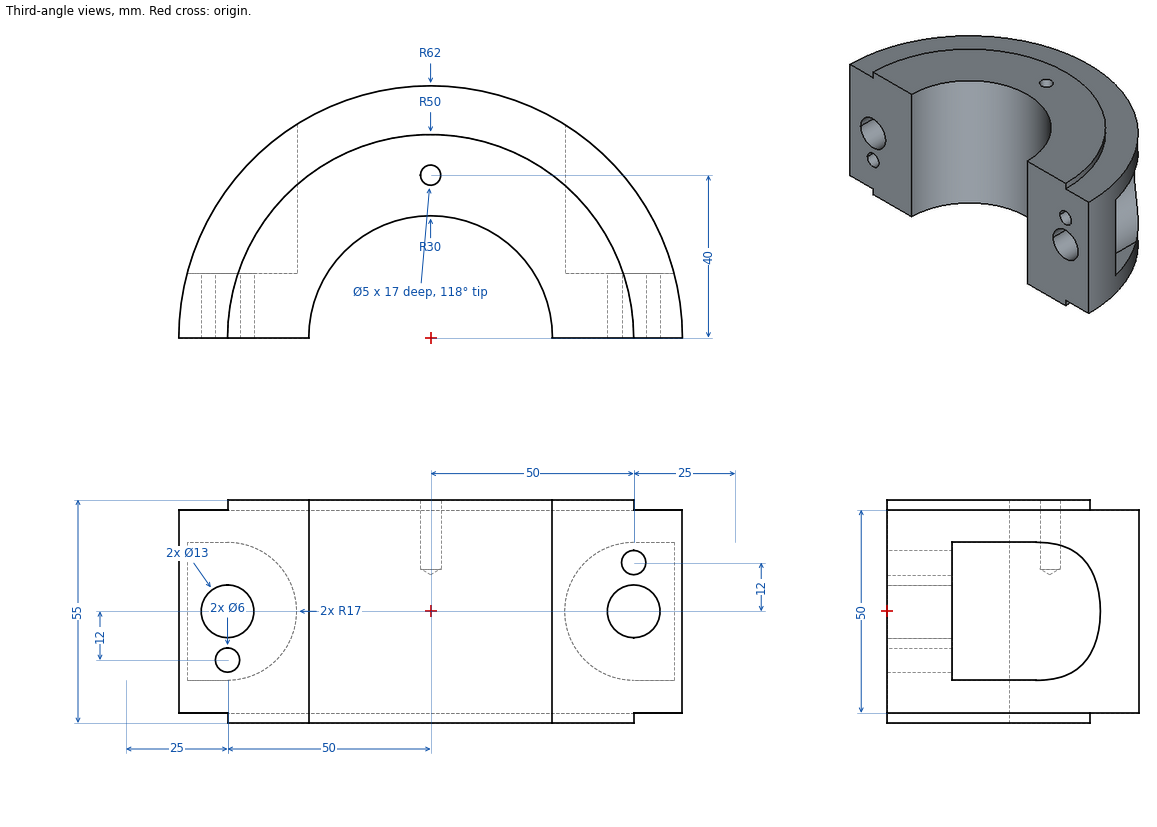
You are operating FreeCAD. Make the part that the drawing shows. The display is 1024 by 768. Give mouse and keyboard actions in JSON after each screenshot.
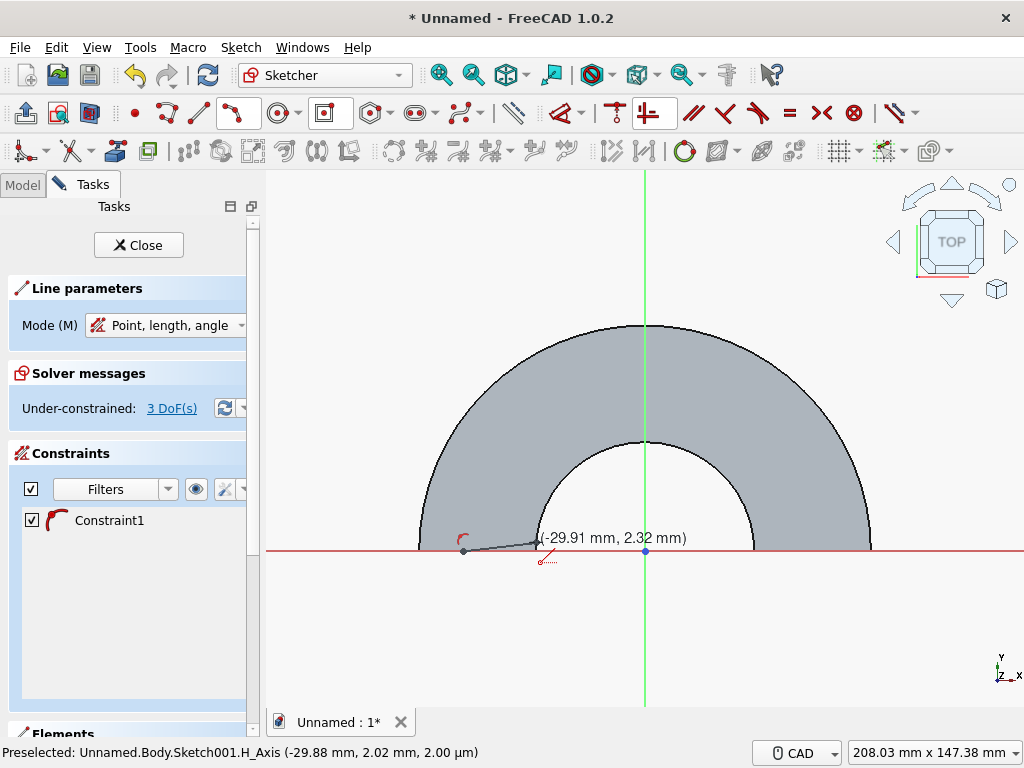
{"action": "left_click", "coordinate": [754, 551]}
{"action": "left_click", "coordinate": [827, 542]}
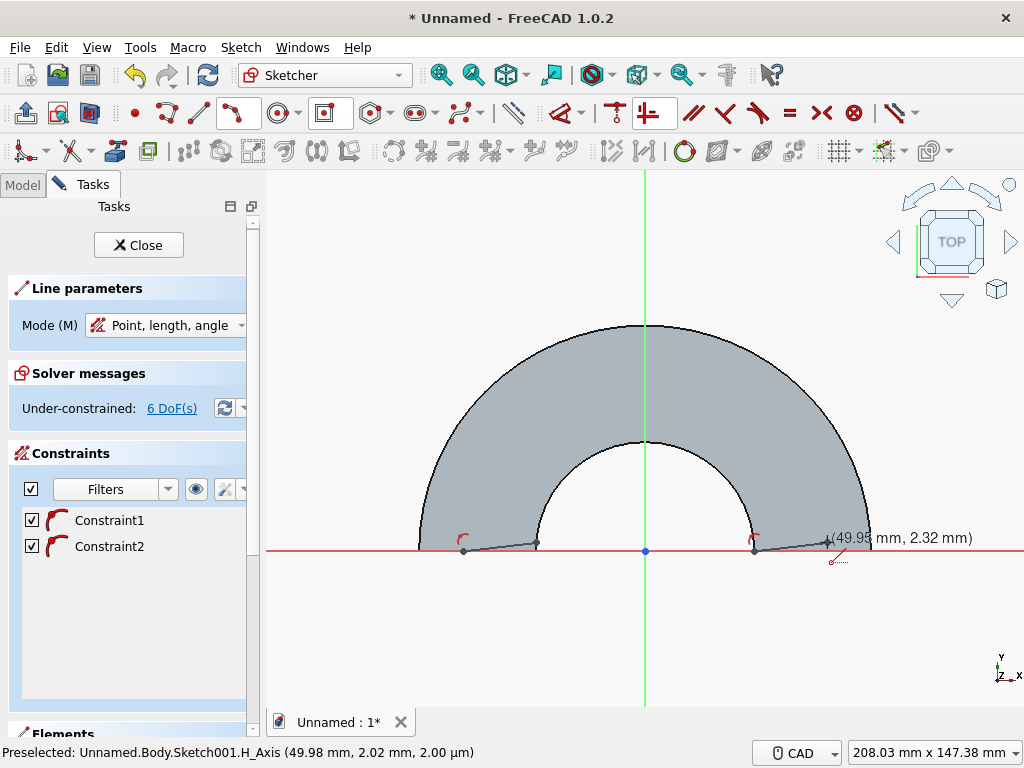
{"action": "left_click", "coordinate": [232, 114]}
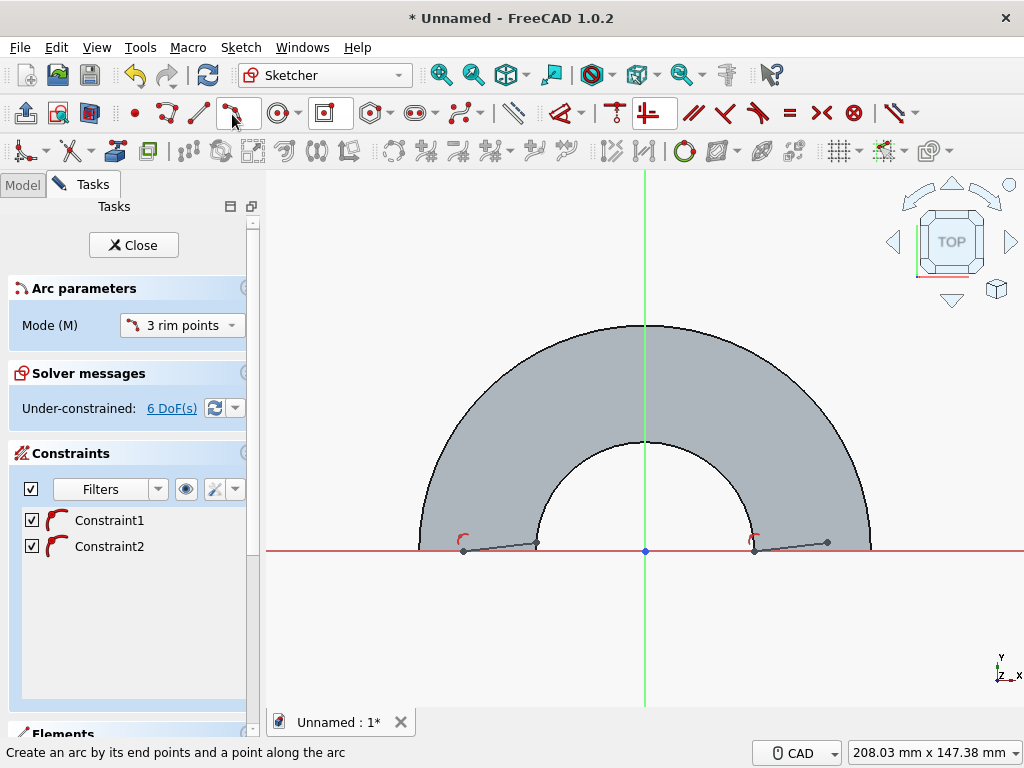
{"action": "left_click", "coordinate": [536, 543]}
{"action": "left_click", "coordinate": [754, 551]}
{"action": "left_click", "coordinate": [679, 447]}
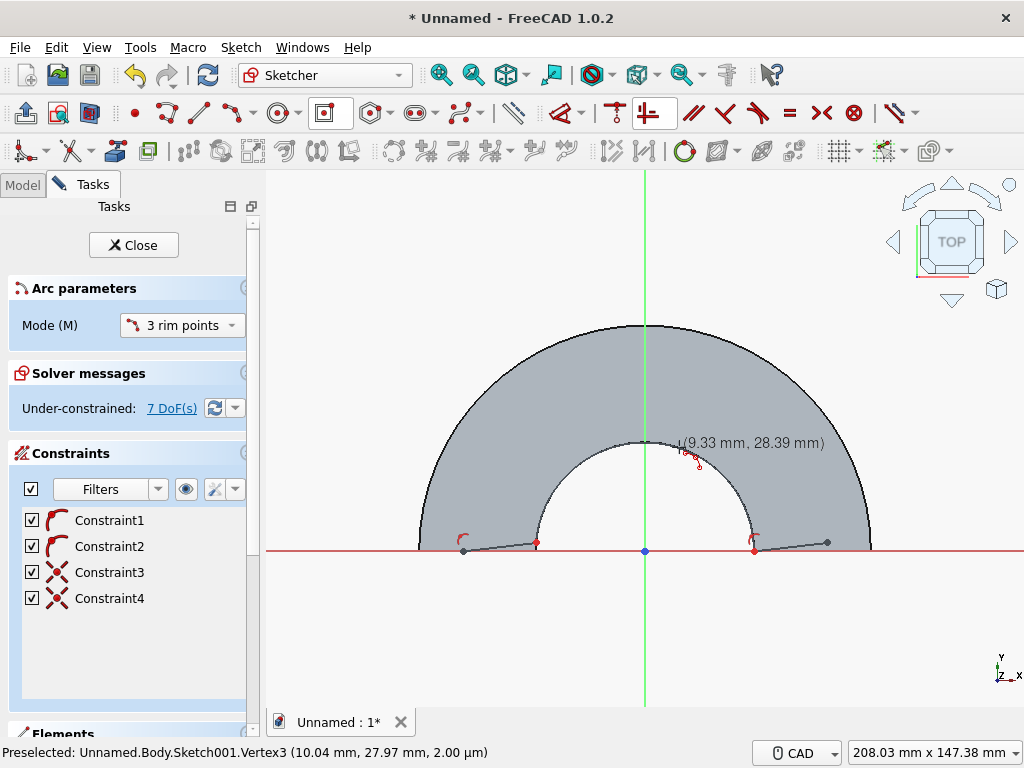
{"action": "left_click", "coordinate": [827, 543]}
{"action": "left_click", "coordinate": [463, 551]}
{"action": "left_click", "coordinate": [701, 378]}
{"action": "key", "text": "Escape"}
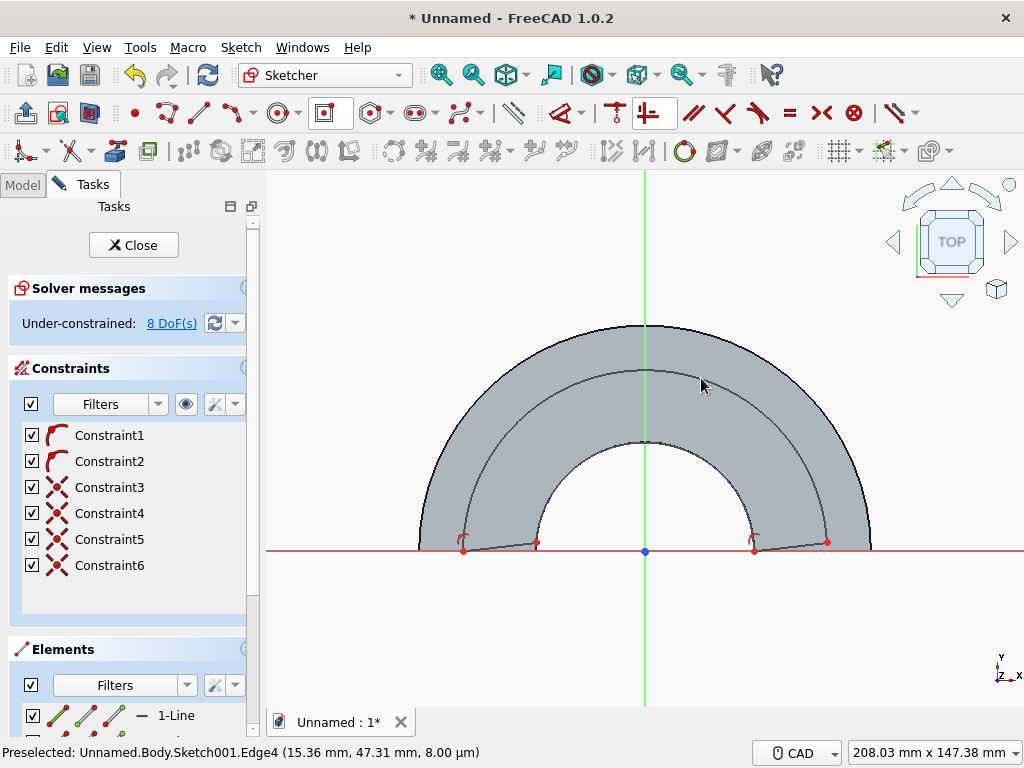
{"action": "left_click", "coordinate": [485, 549]}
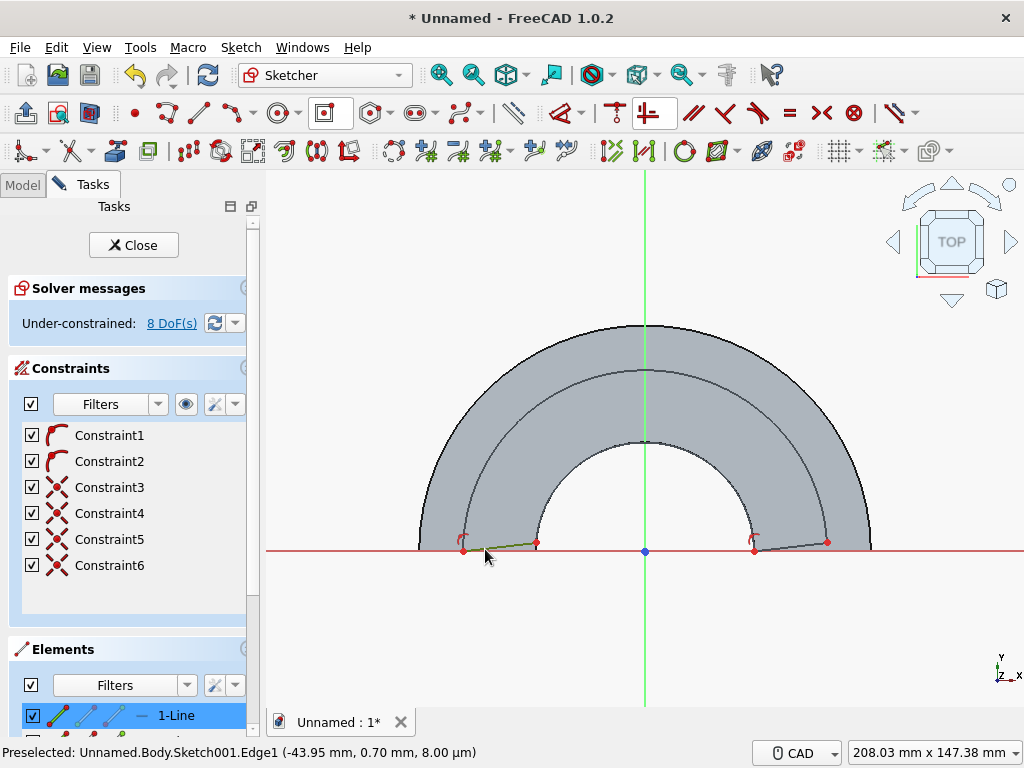
{"action": "key", "text": "h"}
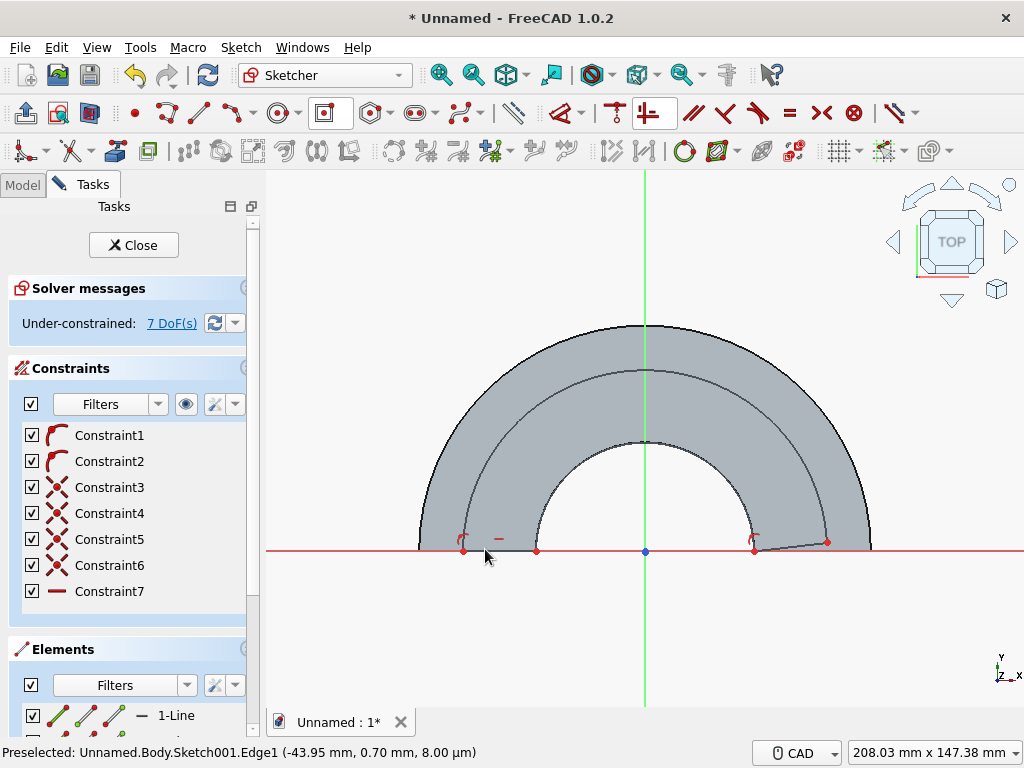
{"action": "left_click", "coordinate": [776, 549]}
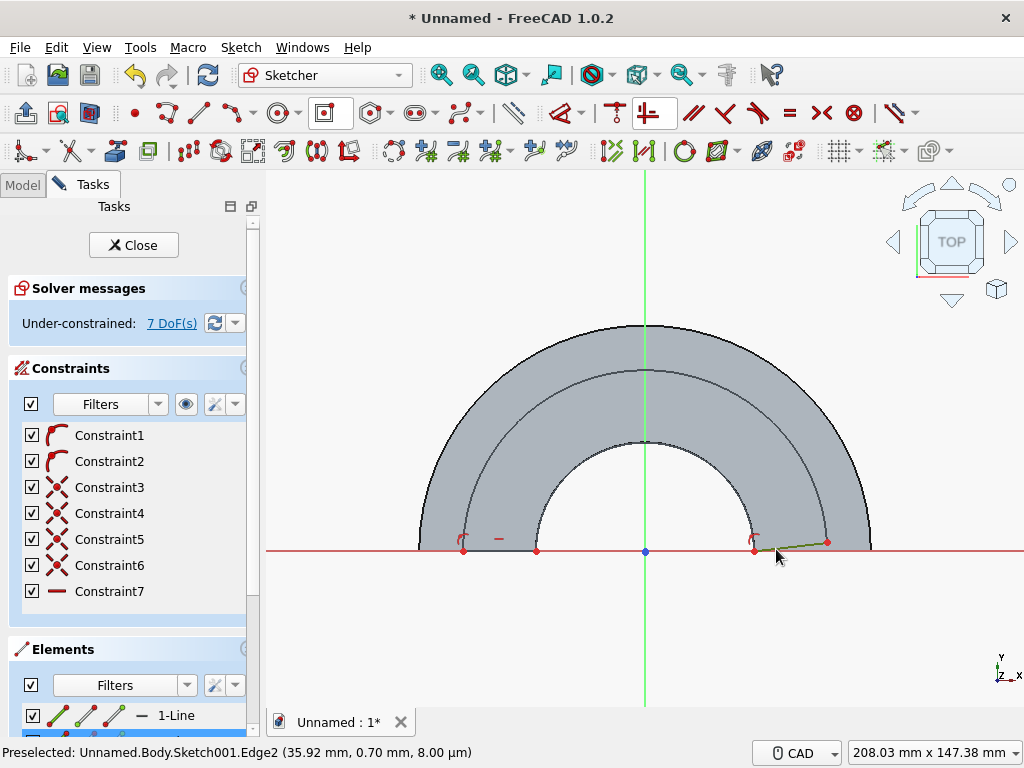
{"action": "key", "text": "h"}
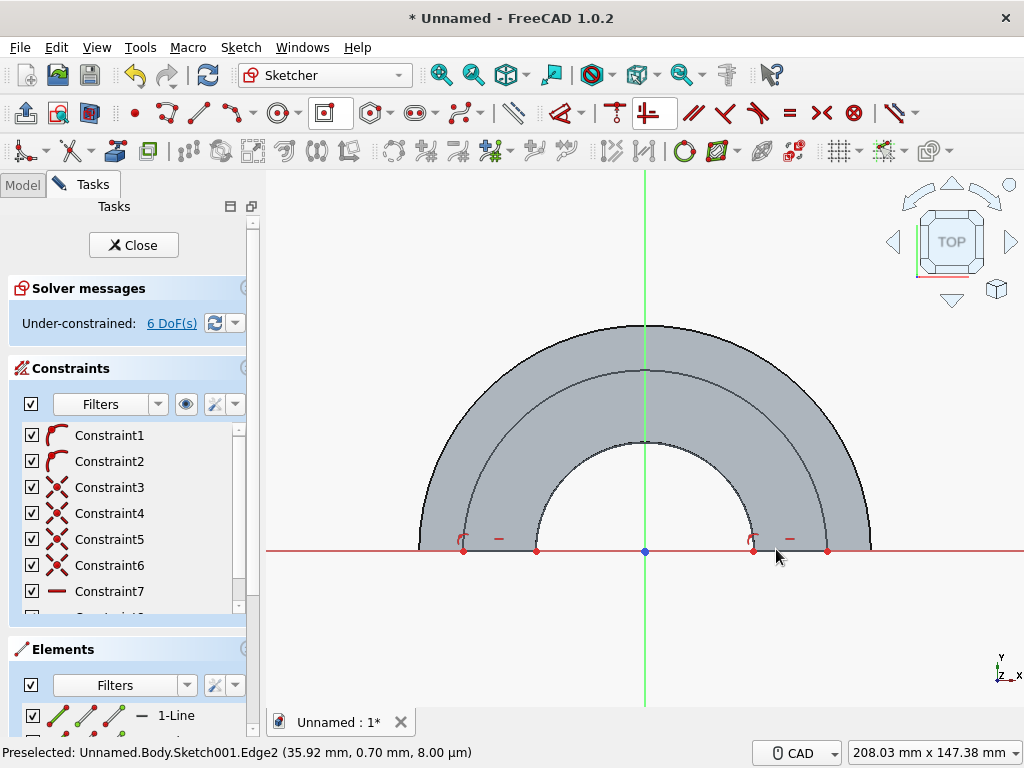
{"action": "left_click", "coordinate": [709, 463]}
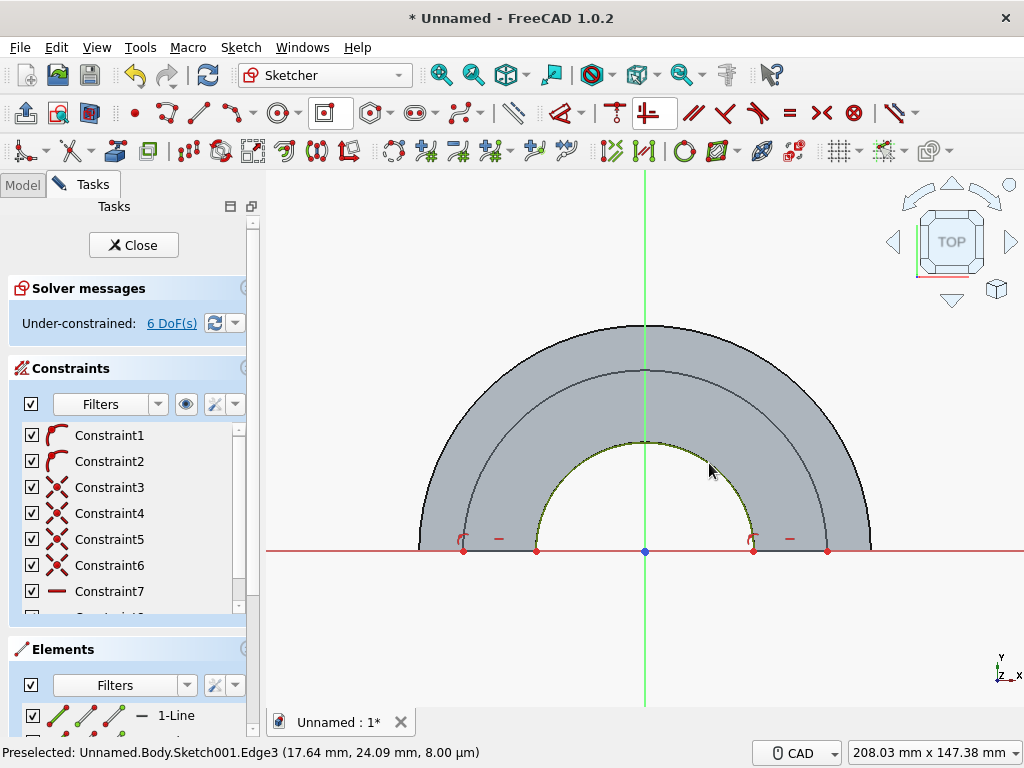
{"action": "left_click", "coordinate": [752, 405]}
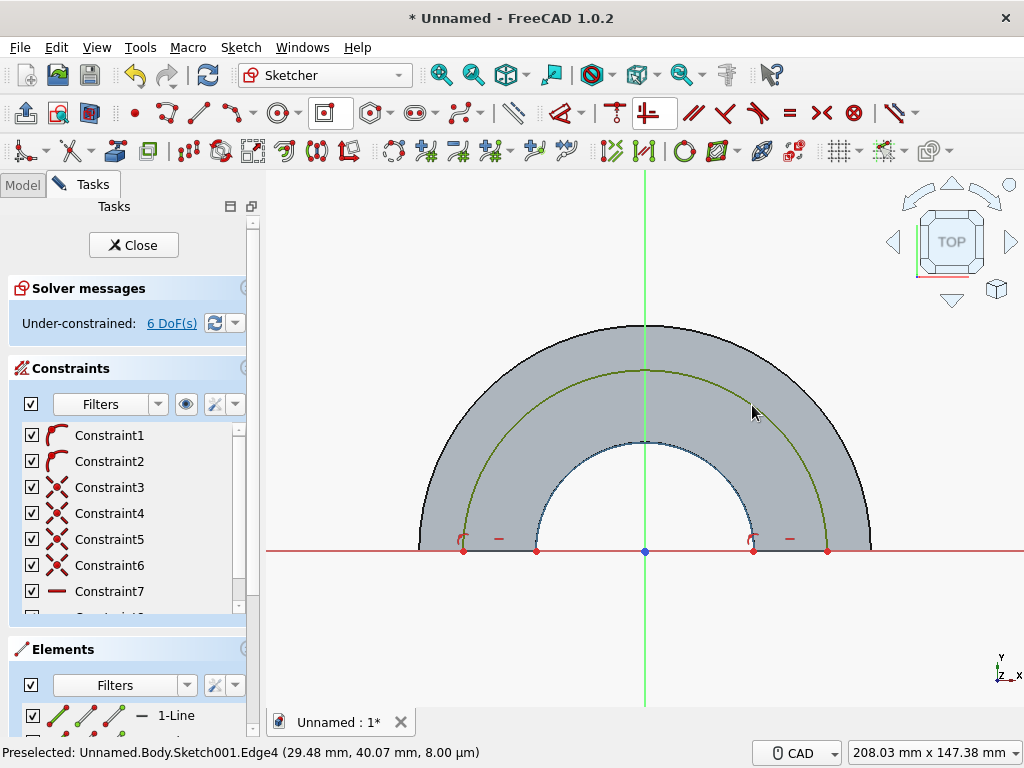
{"action": "left_click", "coordinate": [616, 114]}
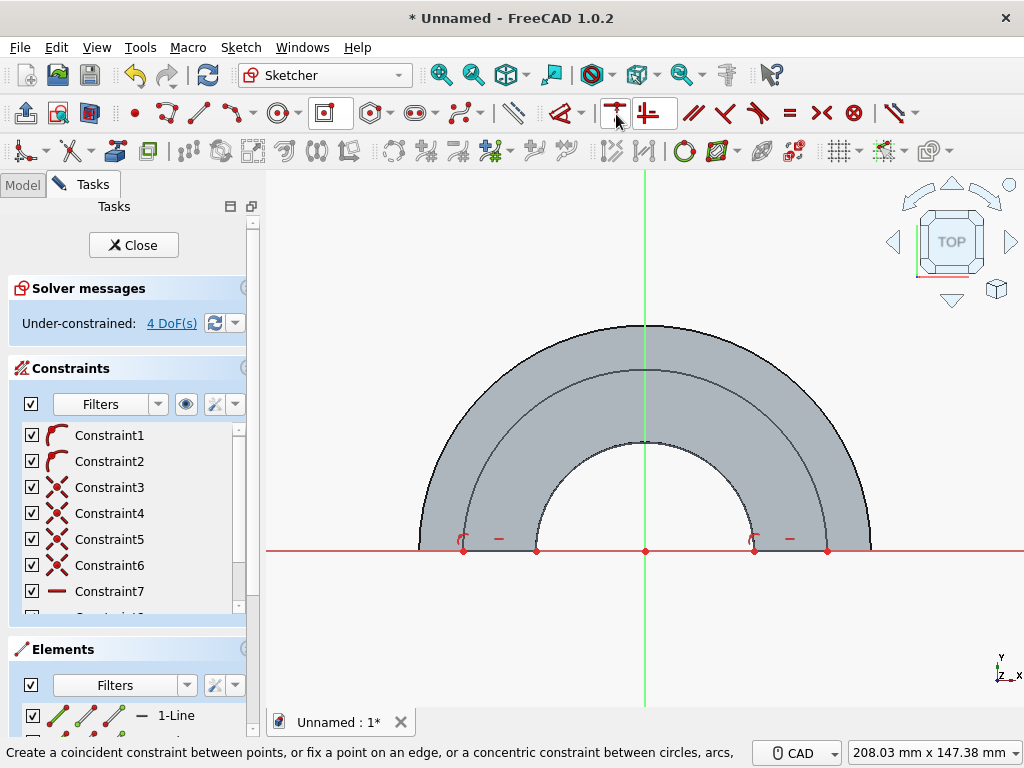
{"action": "left_click_drag", "start_coordinate": [635, 541], "coordinate": [655, 562]}